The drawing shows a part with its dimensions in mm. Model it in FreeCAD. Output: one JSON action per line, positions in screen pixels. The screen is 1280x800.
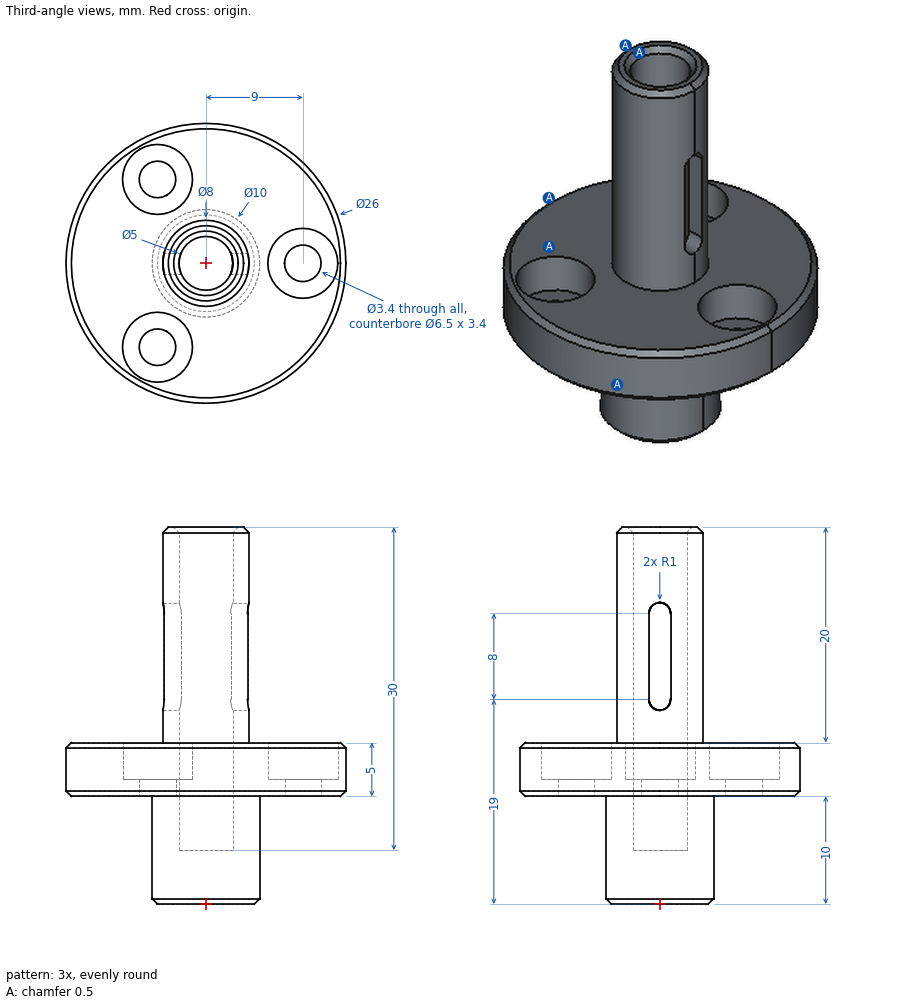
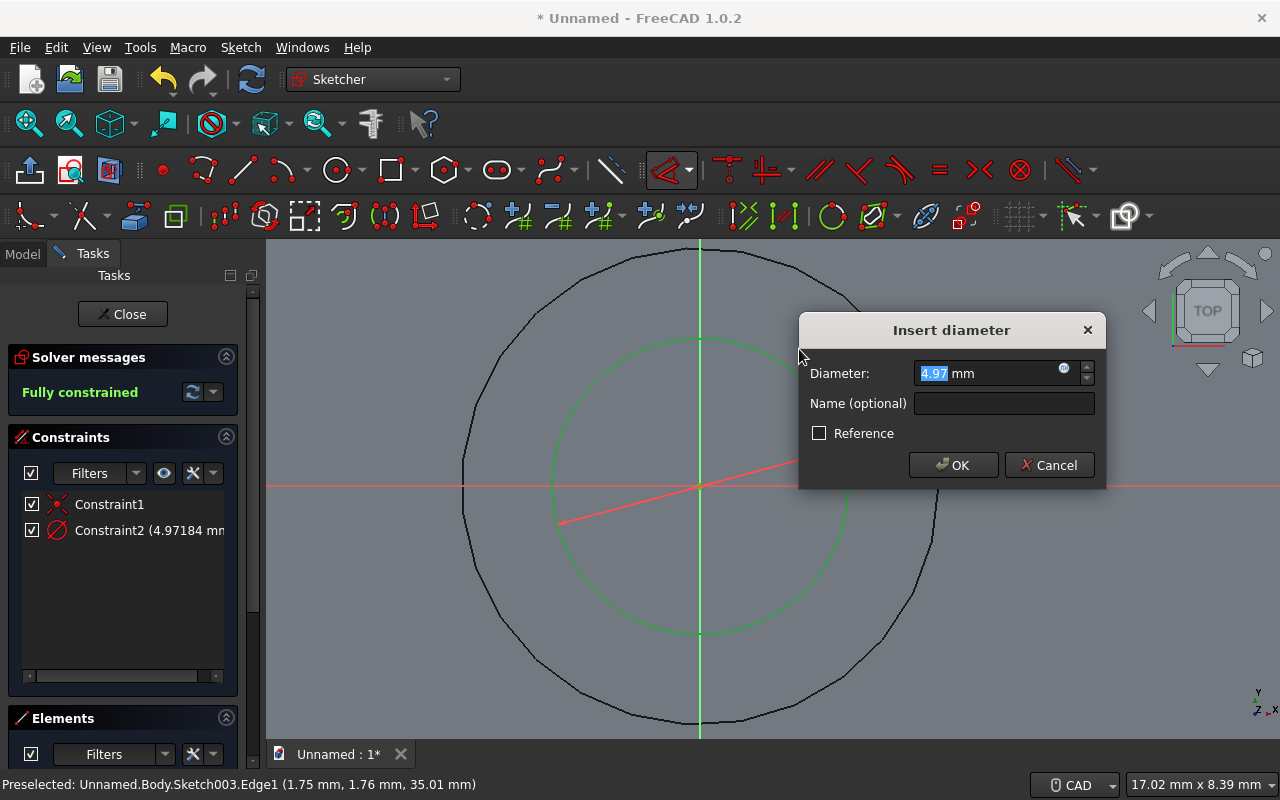
{"action": "type", "text": "5"}
{"action": "key", "text": "Return"}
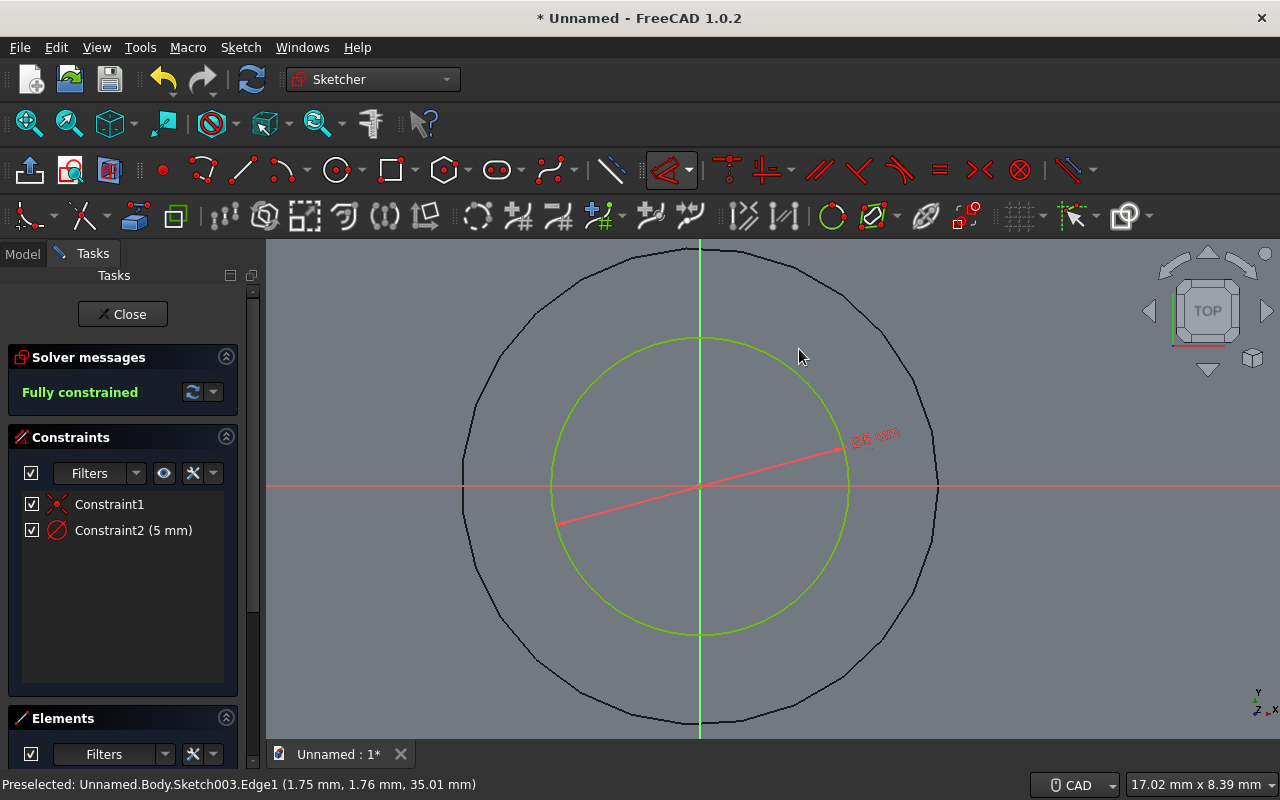
{"action": "left_click", "coordinate": [123, 314]}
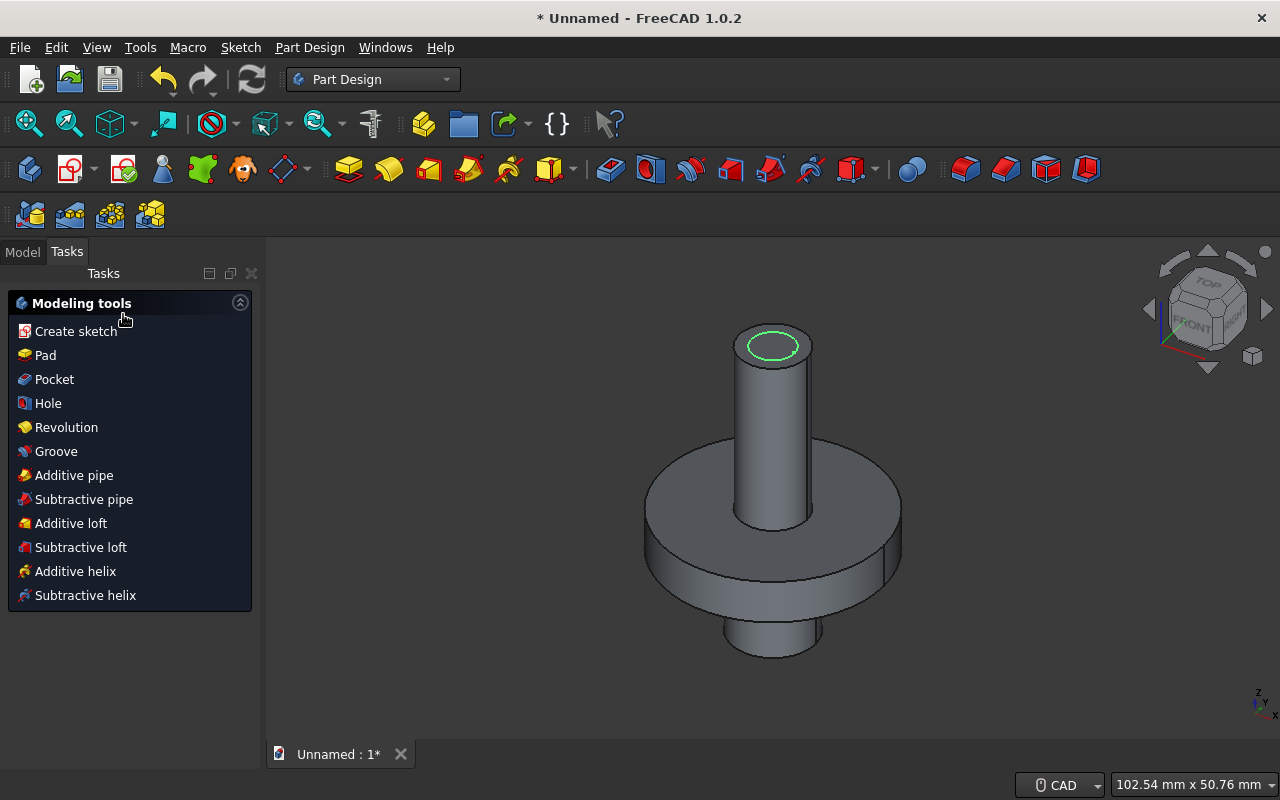
{"action": "left_click", "coordinate": [612, 170]}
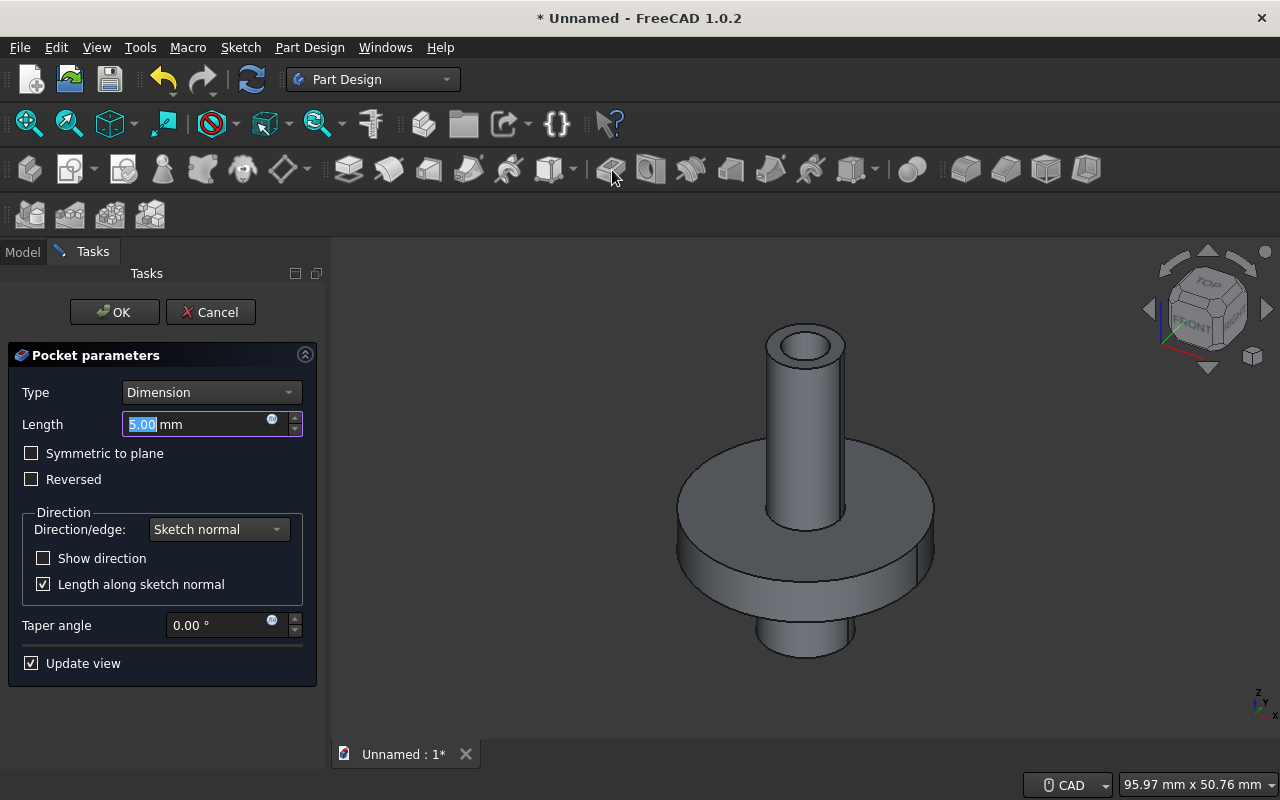
{"action": "type", "text": "30"}
{"action": "key", "text": "Tab"}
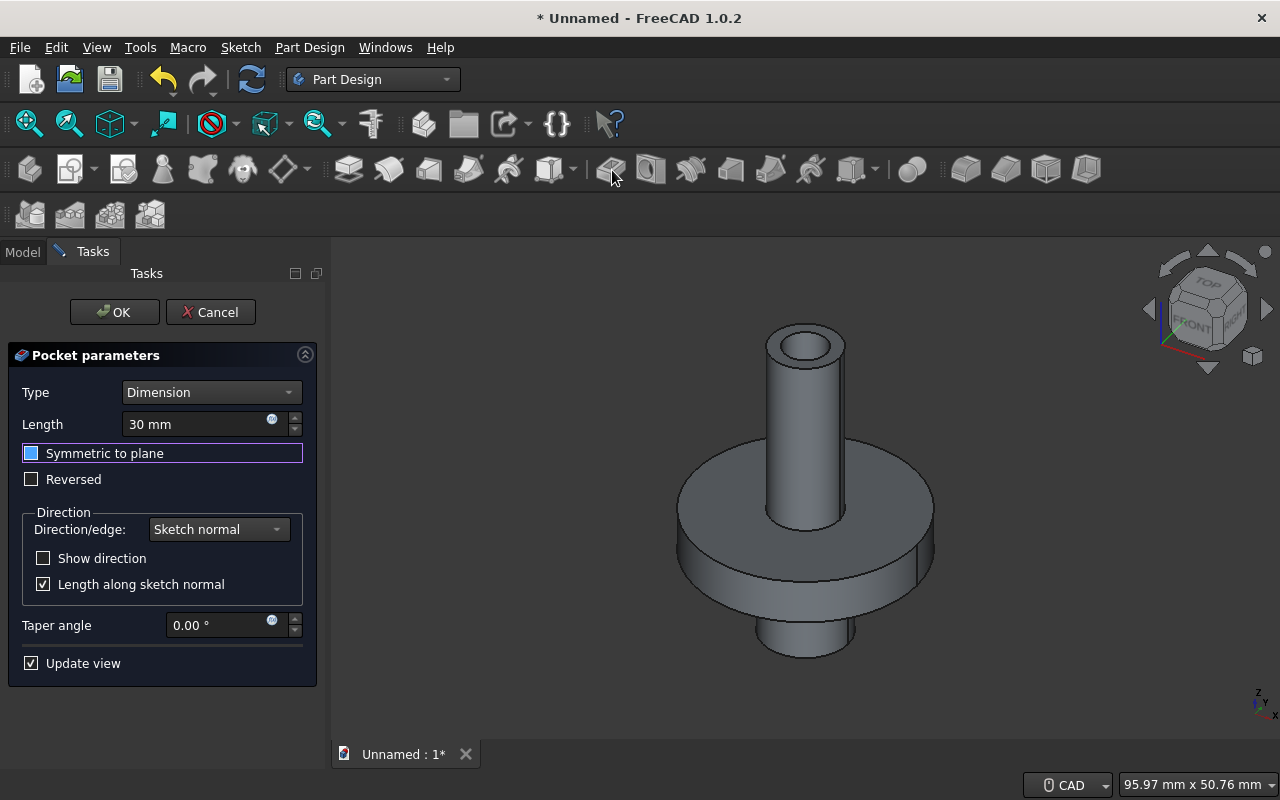
{"action": "left_click", "coordinate": [115, 312]}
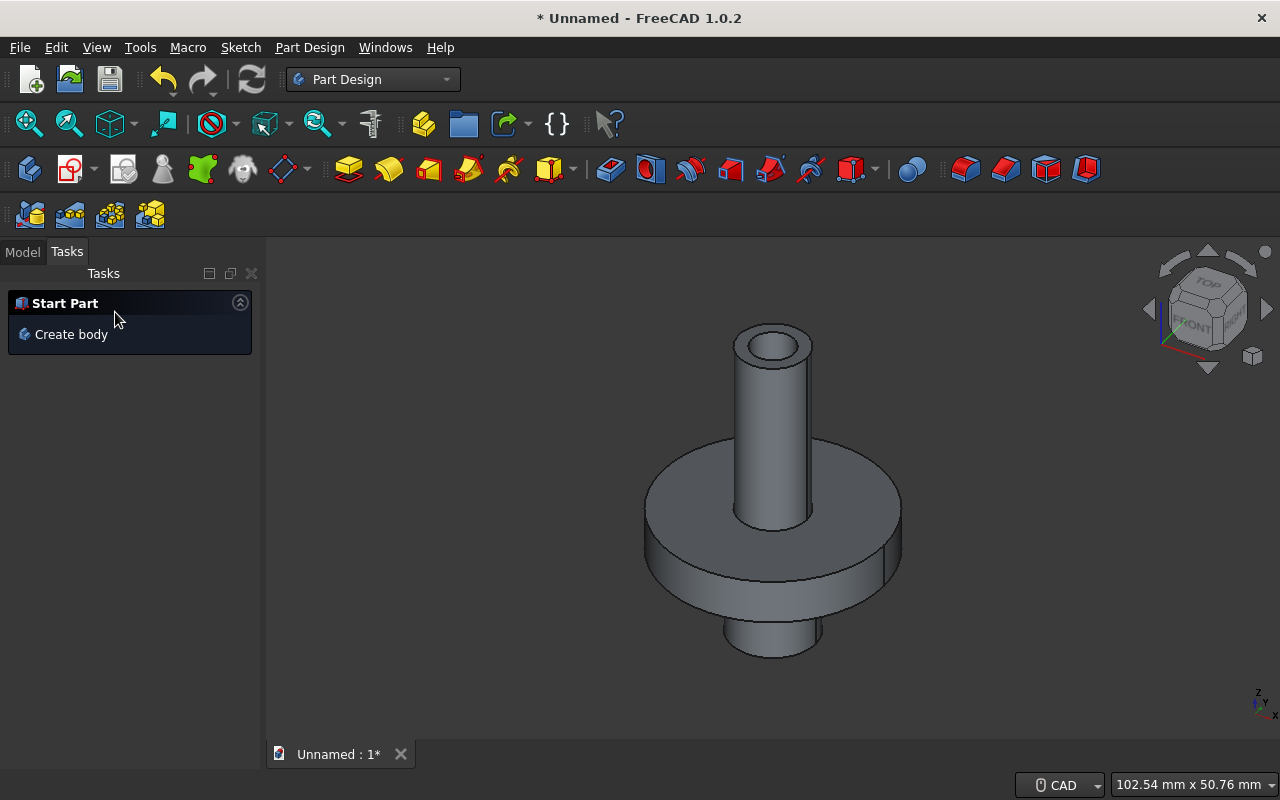
{"action": "left_click", "coordinate": [768, 554]}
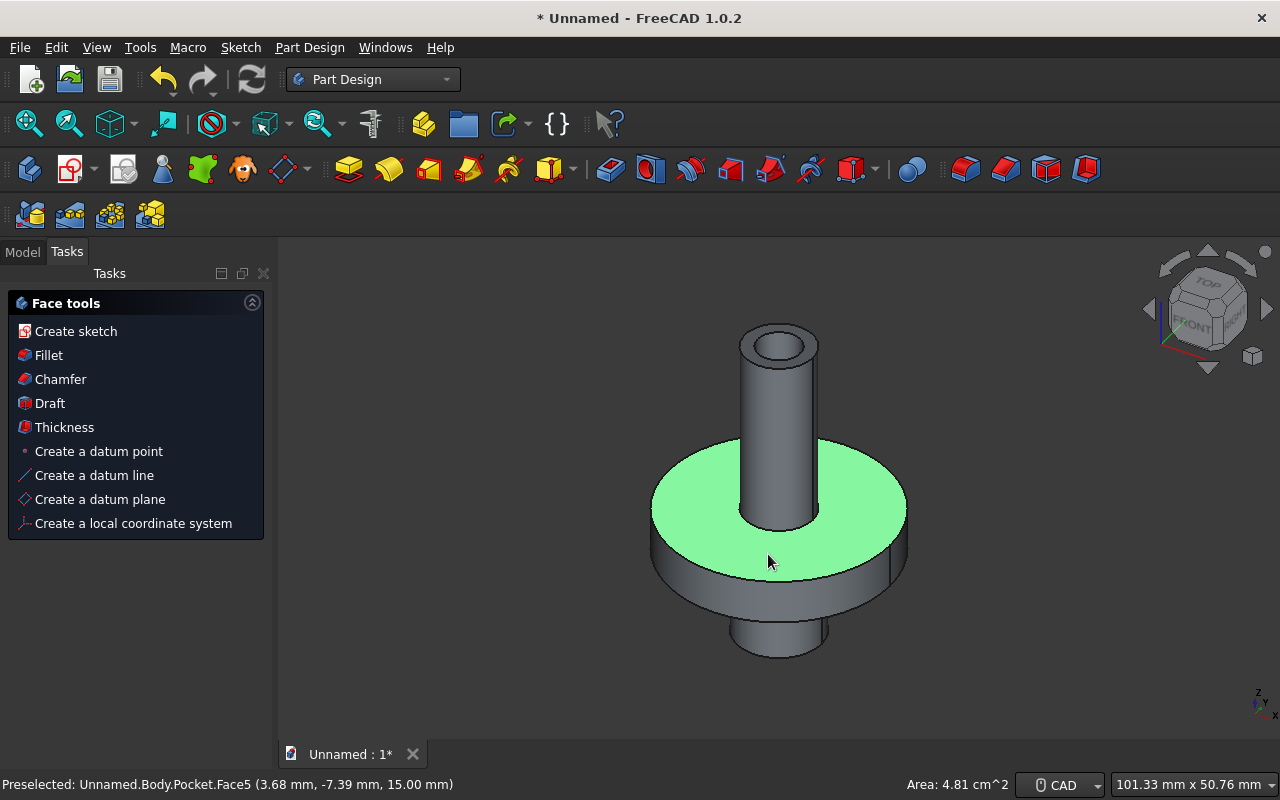
{"action": "left_click", "coordinate": [70, 170]}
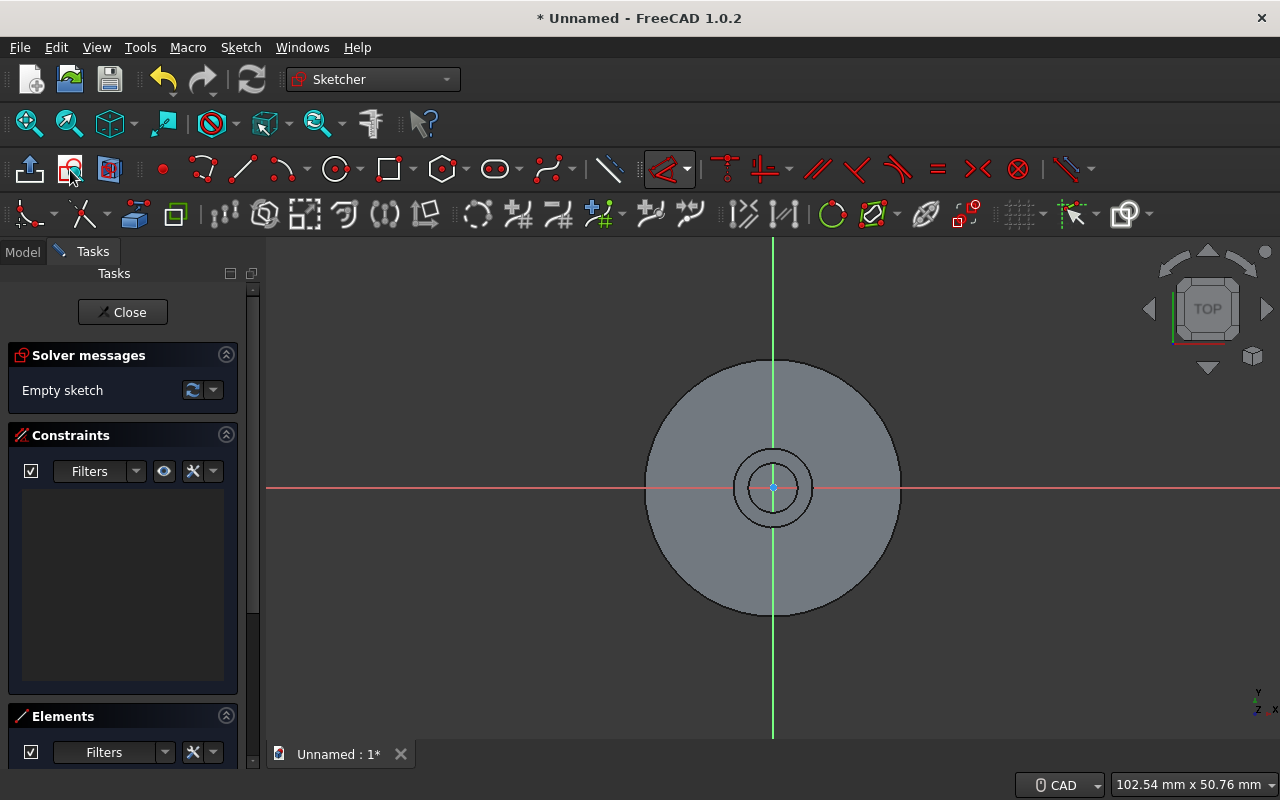
{"action": "left_click", "coordinate": [110, 170]}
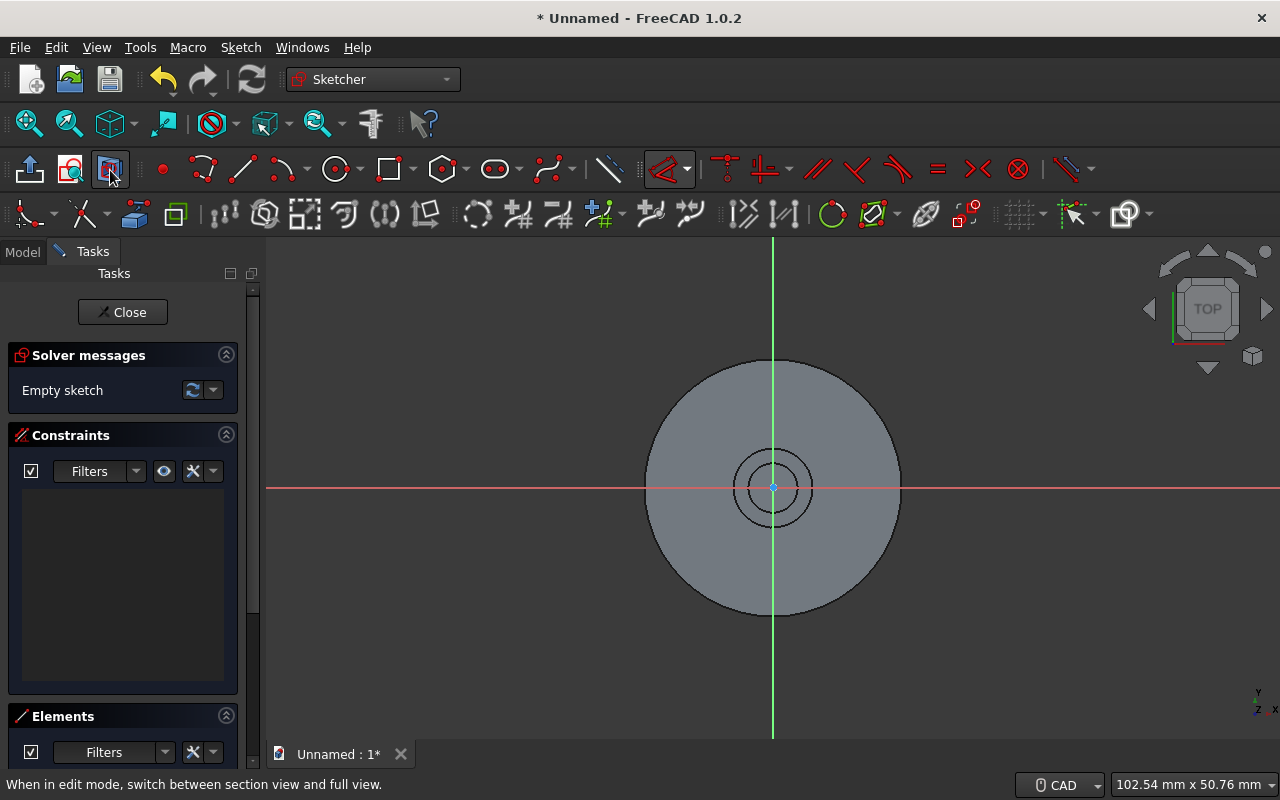
{"action": "scroll", "coordinate": [882, 488], "scroll_direction": "up", "scroll_amount": 11}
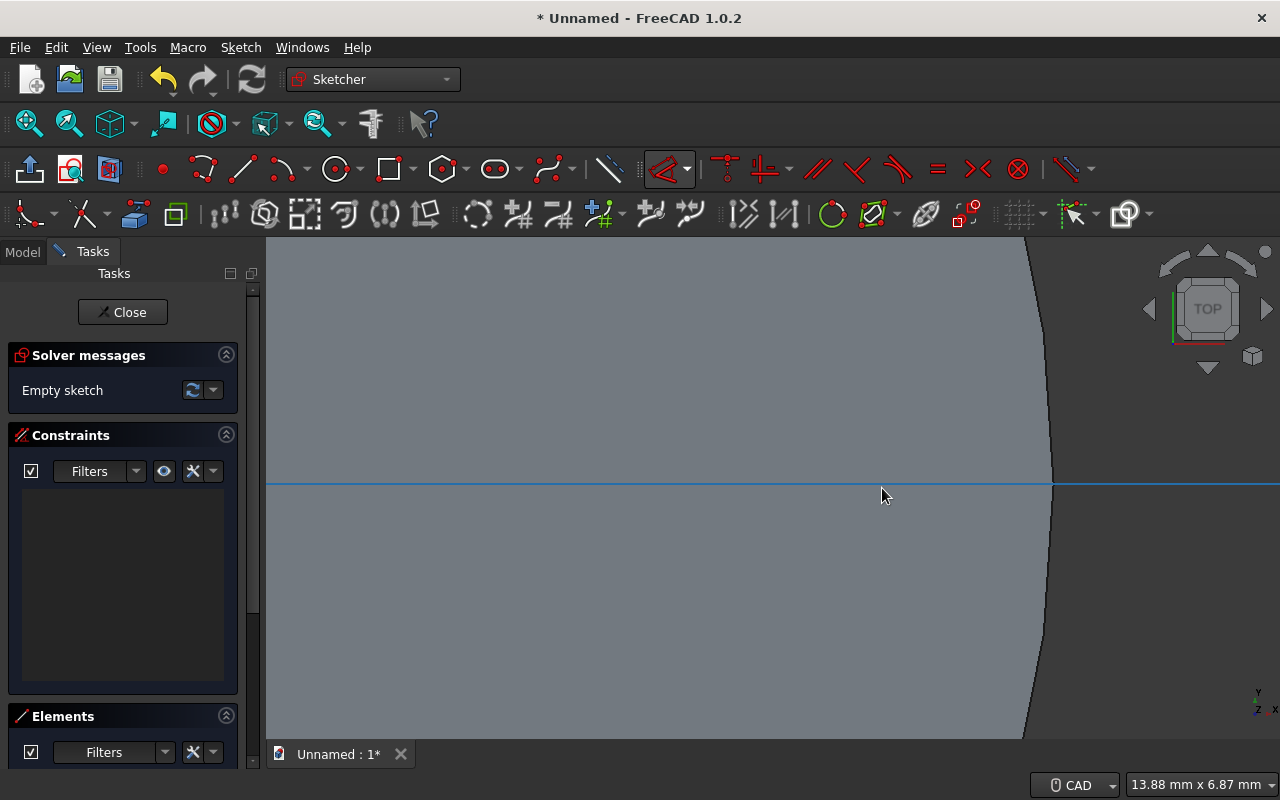
{"action": "left_click", "coordinate": [336, 170]}